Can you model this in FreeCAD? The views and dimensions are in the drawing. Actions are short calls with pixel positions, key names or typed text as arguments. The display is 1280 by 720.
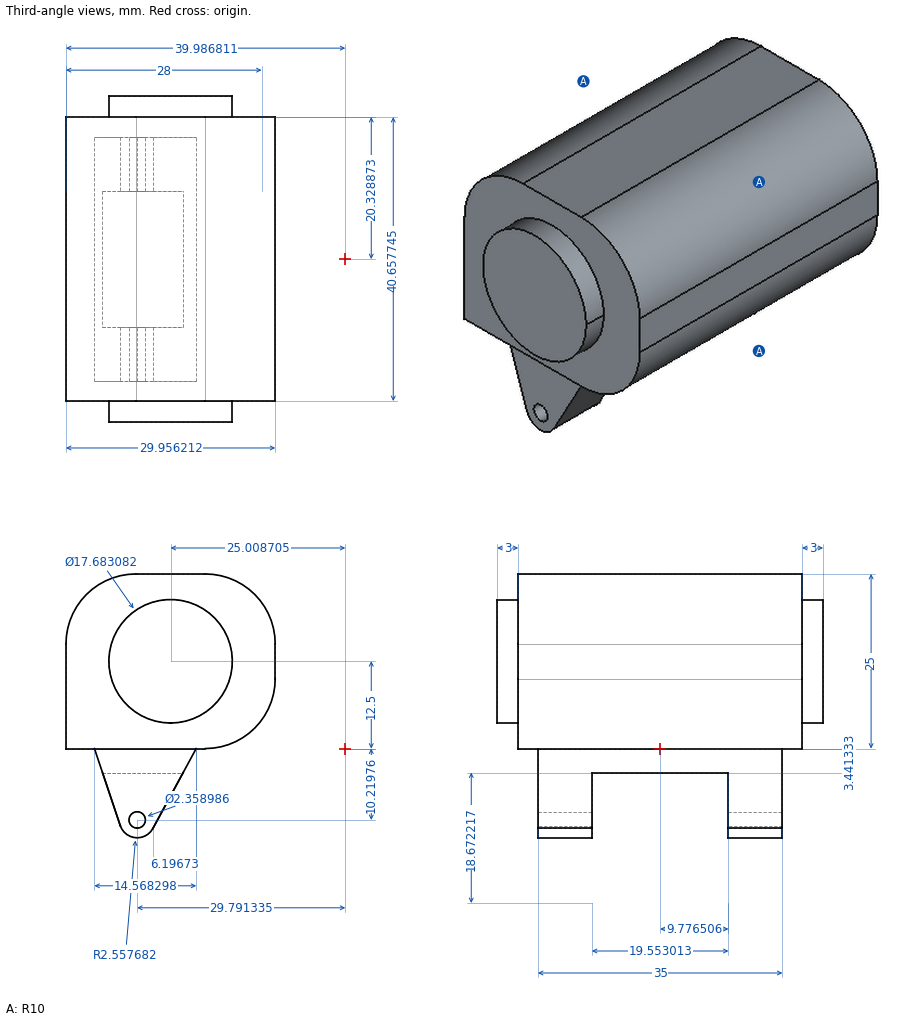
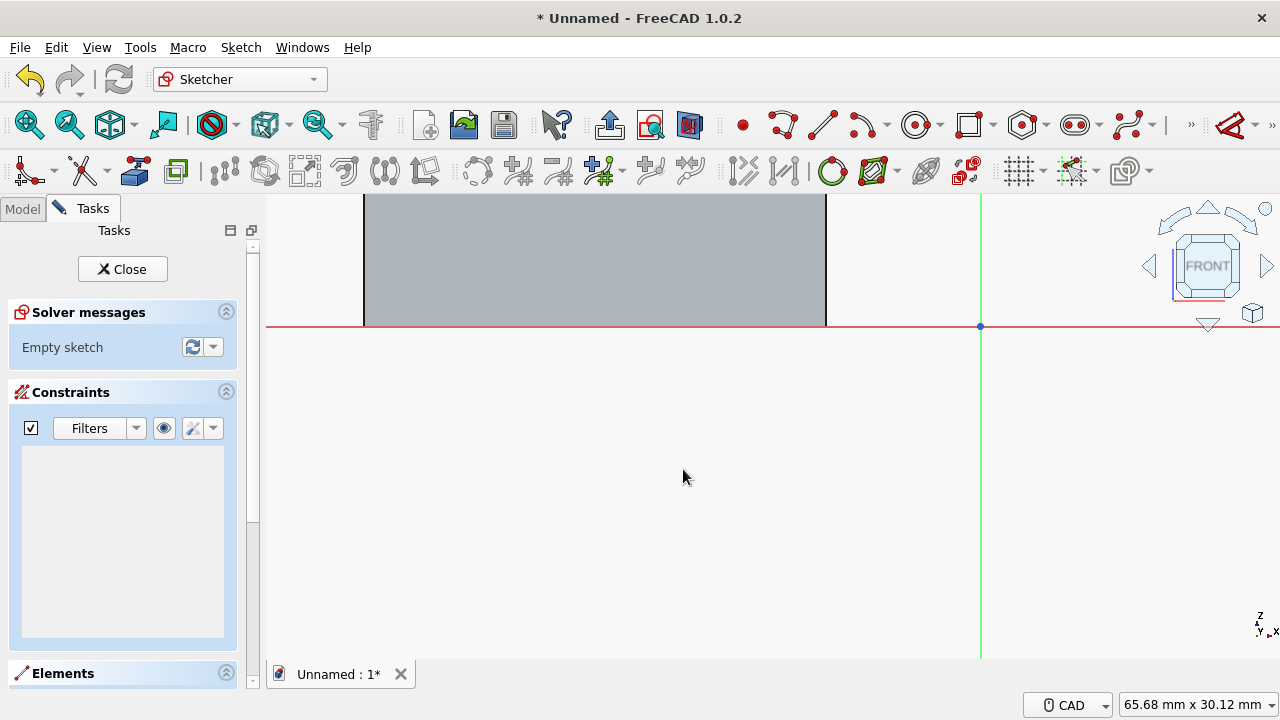
click(784, 126)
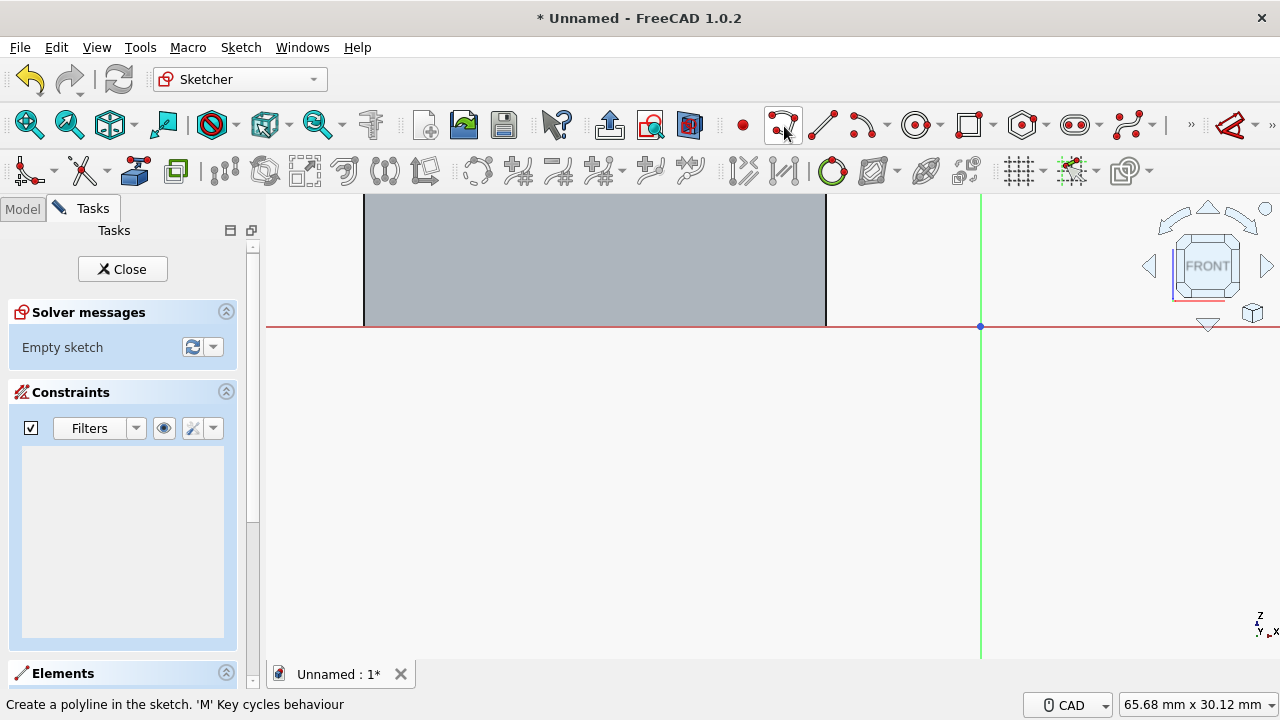
click(556, 503)
click(651, 327)
click(426, 336)
click(483, 497)
right_click(483, 497)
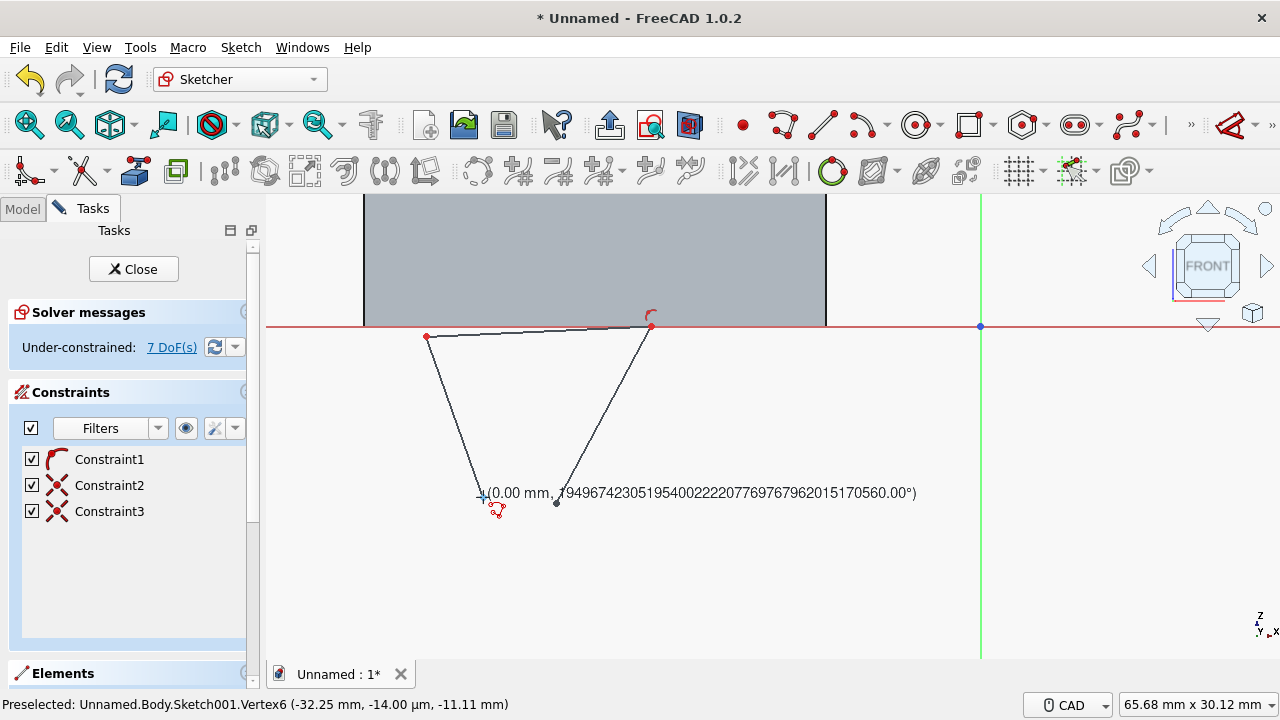
click(890, 126)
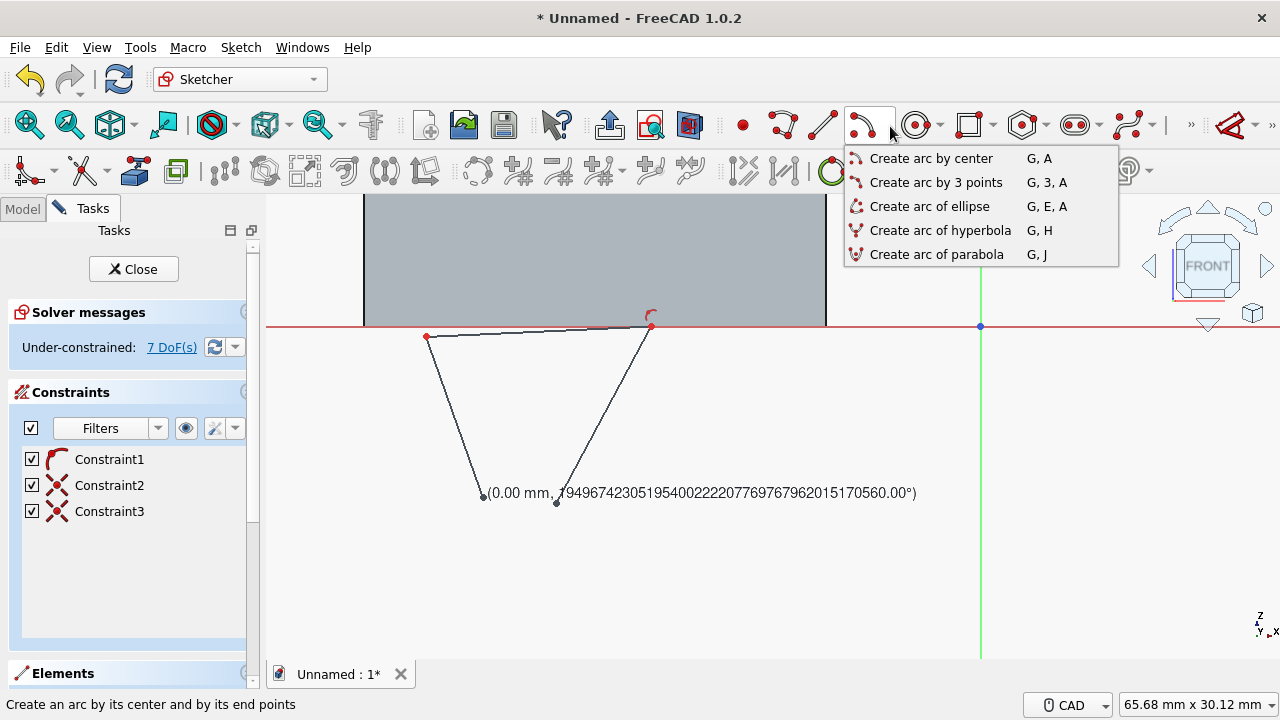
click(982, 182)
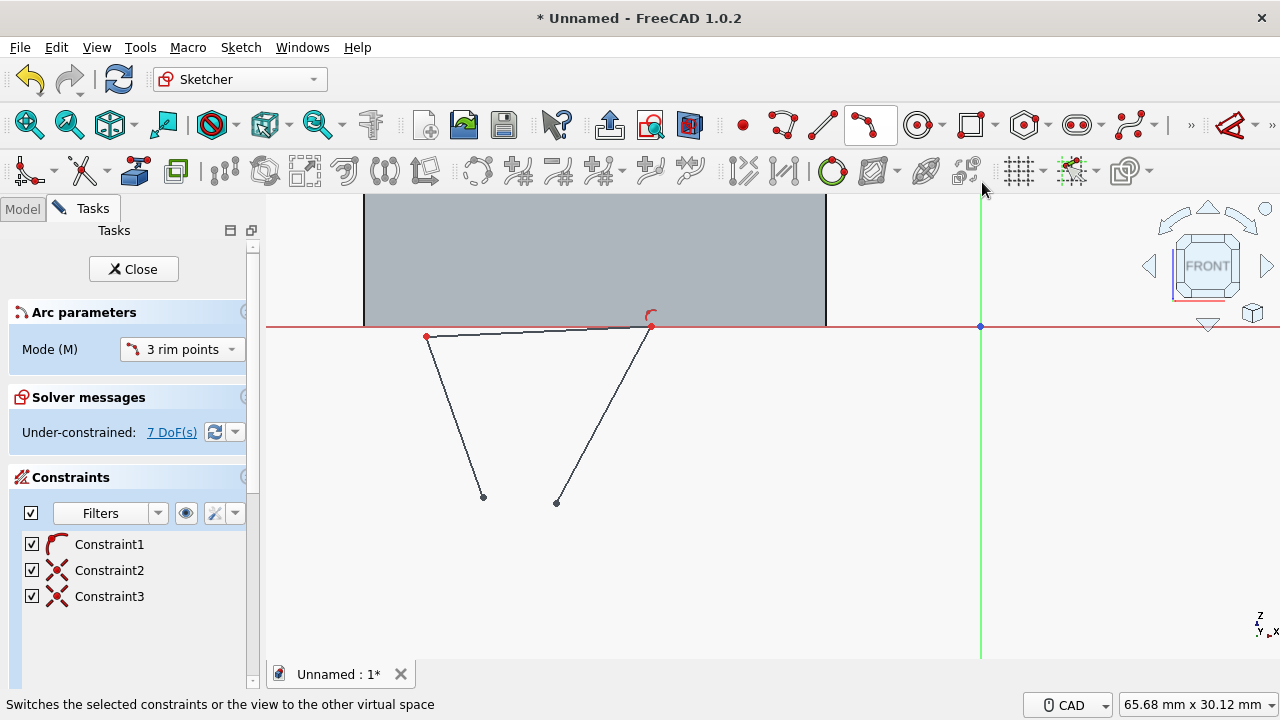
click(483, 498)
click(556, 504)
click(518, 524)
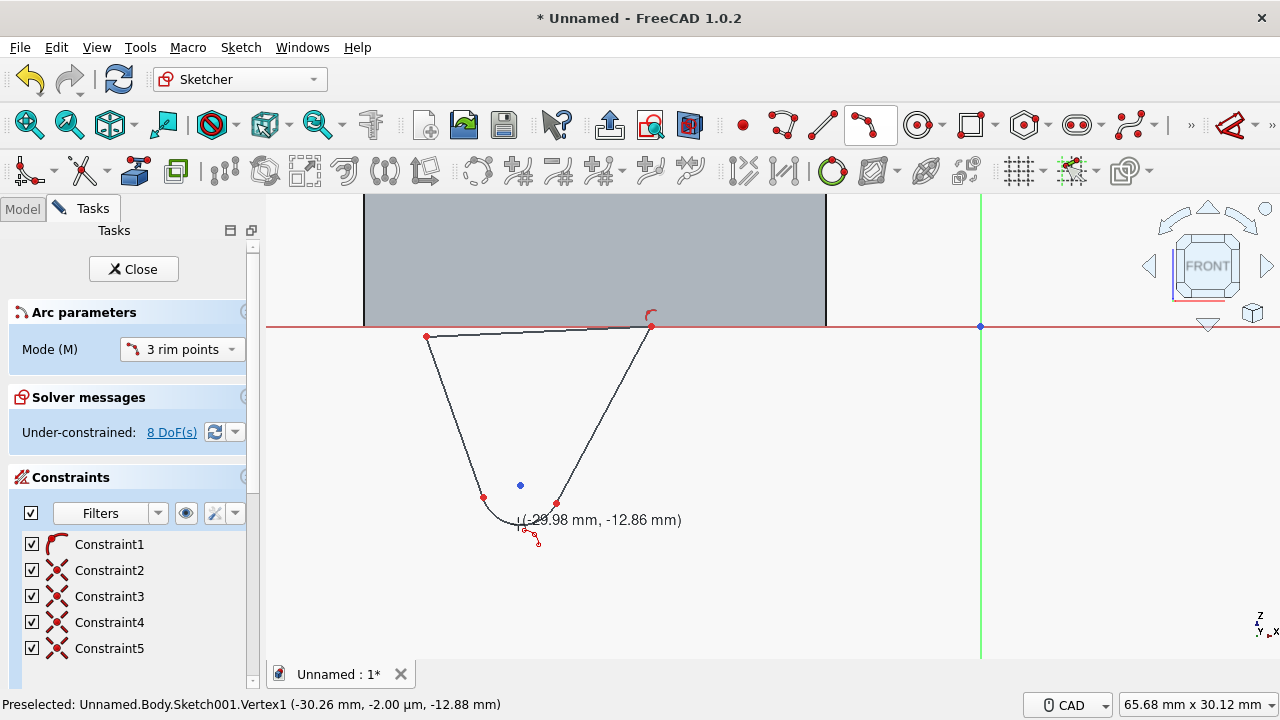
click(918, 126)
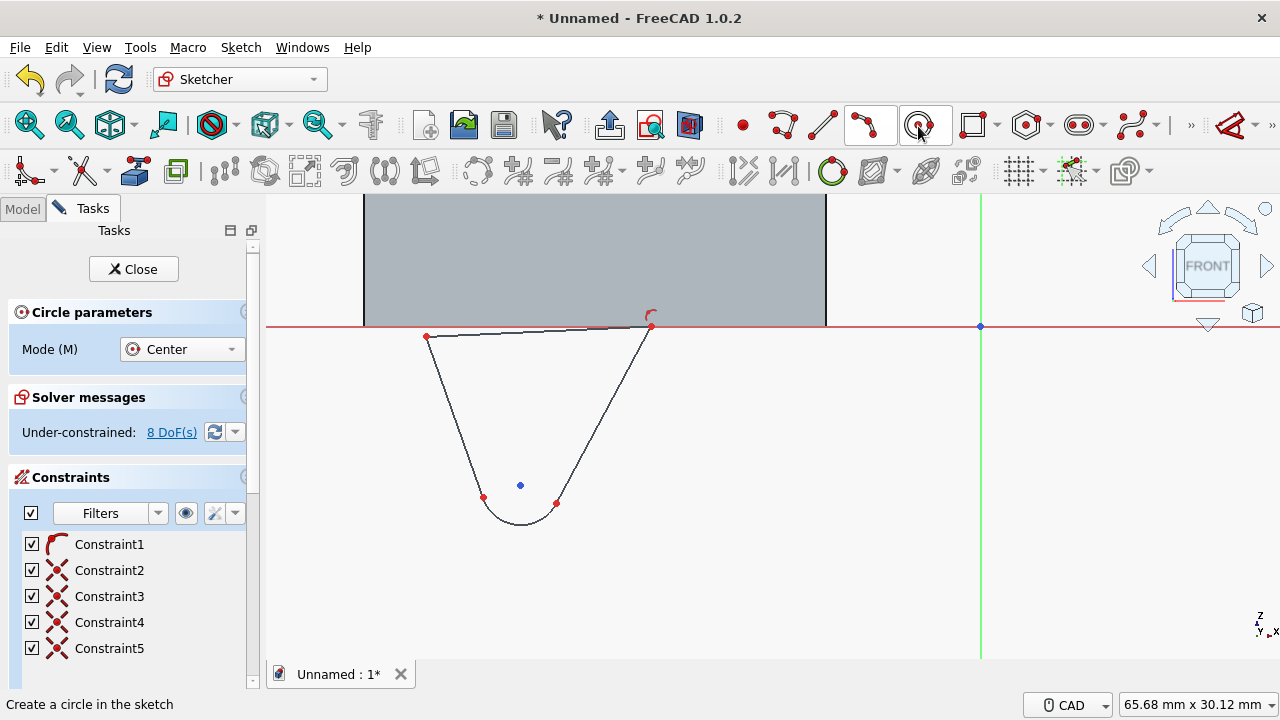
scroll(521, 484, up, 2)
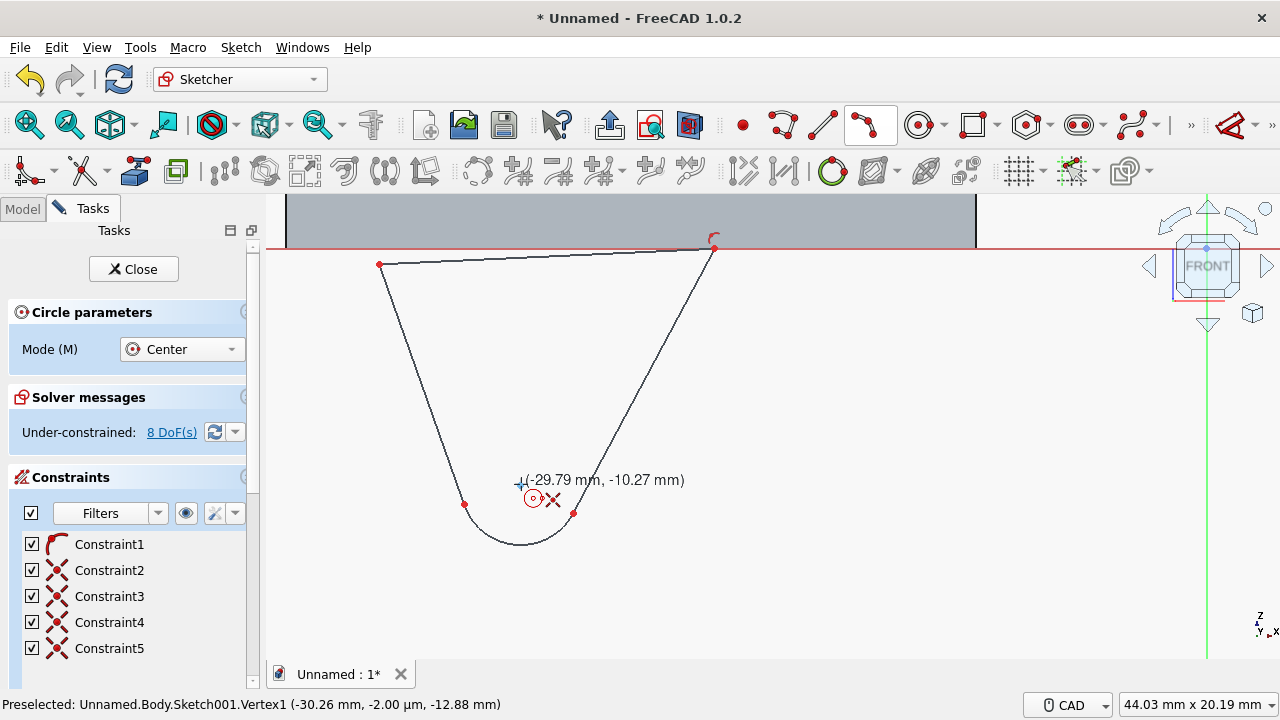
click(521, 484)
move(540, 465)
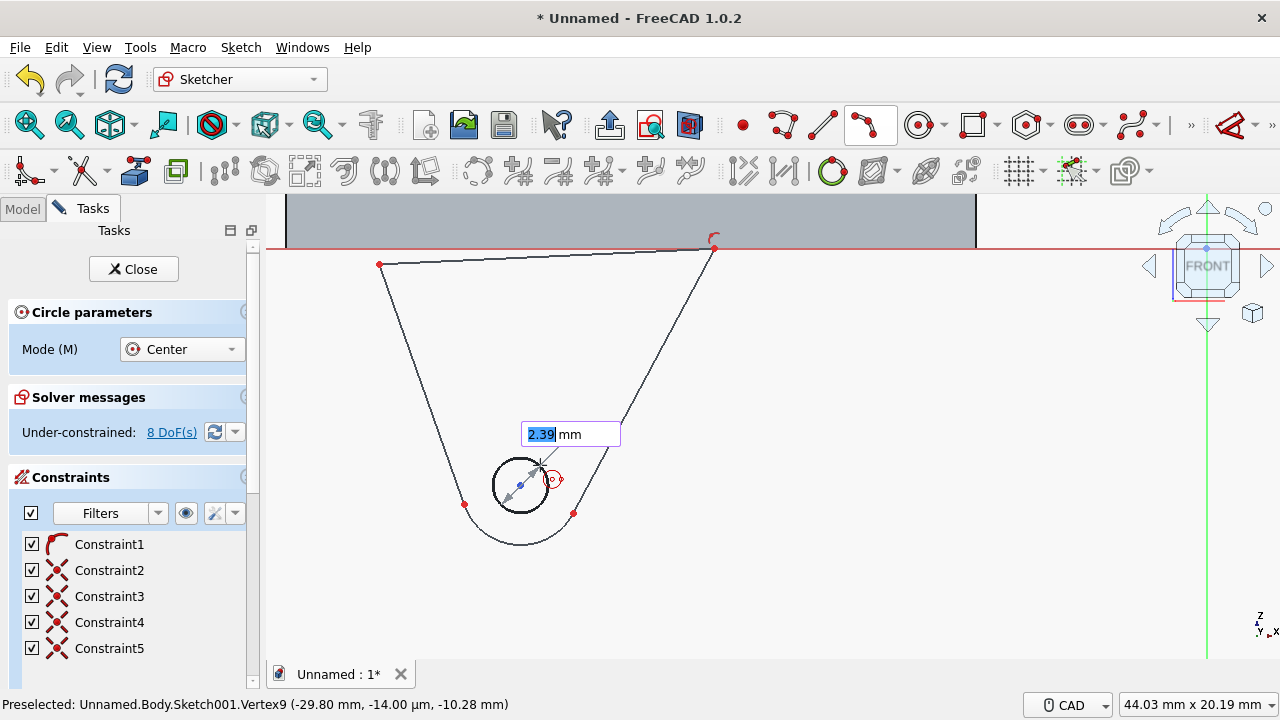
text(2.358986)
key(Return)
key(Escape)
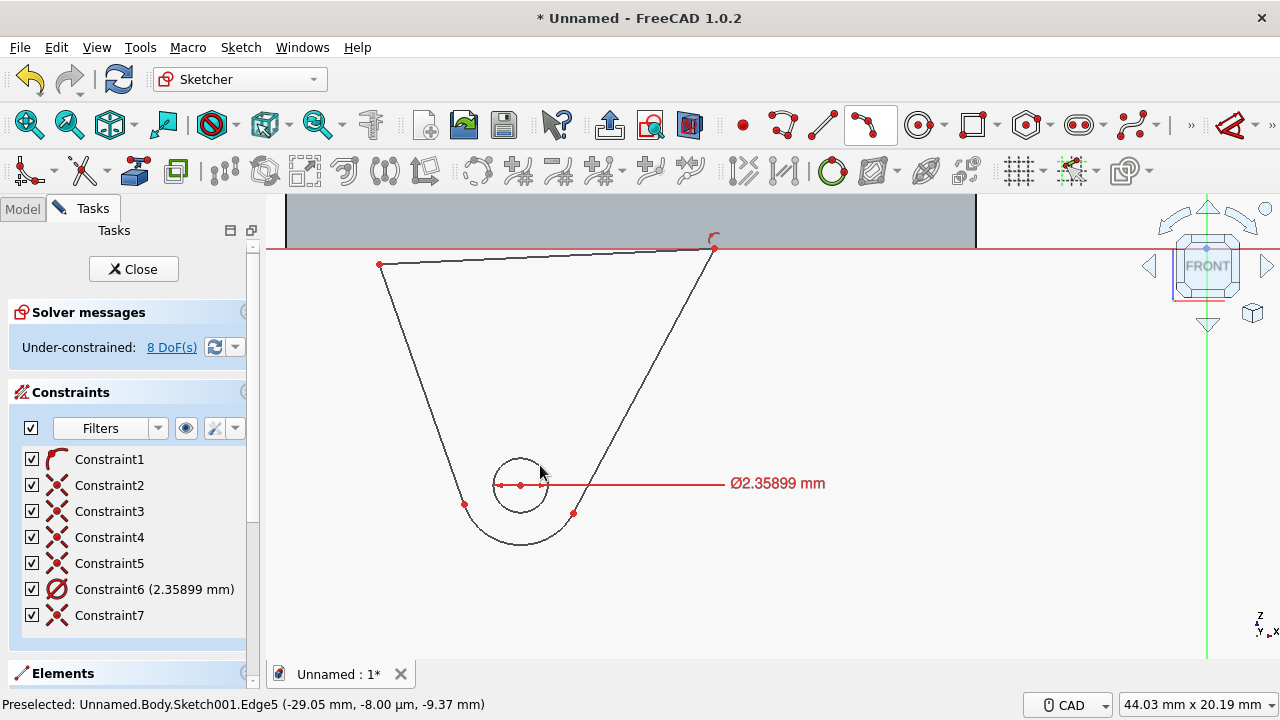
click(616, 434)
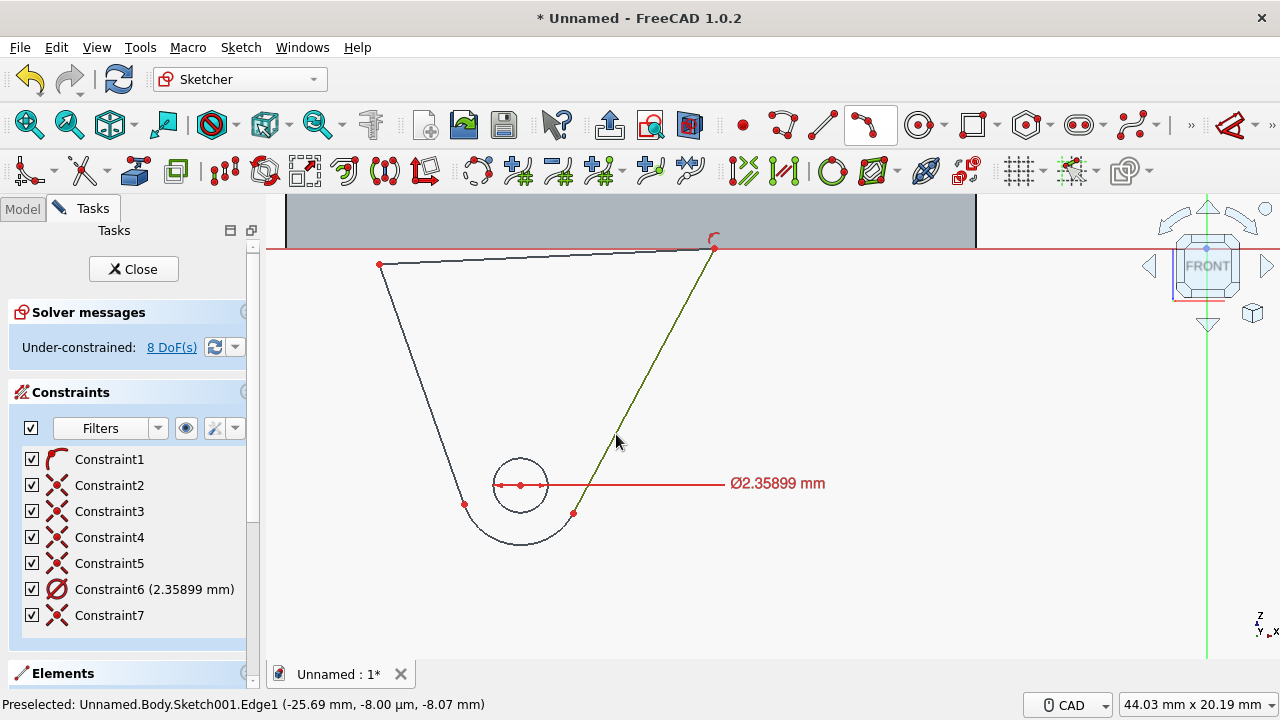
click(490, 536)